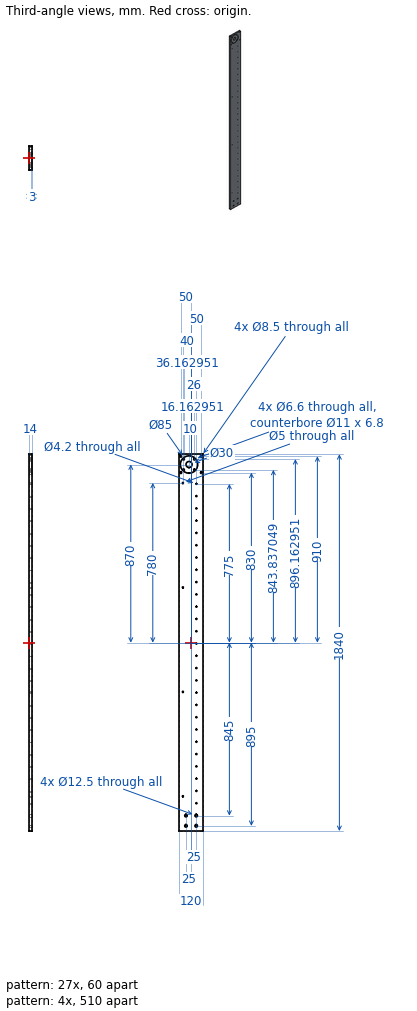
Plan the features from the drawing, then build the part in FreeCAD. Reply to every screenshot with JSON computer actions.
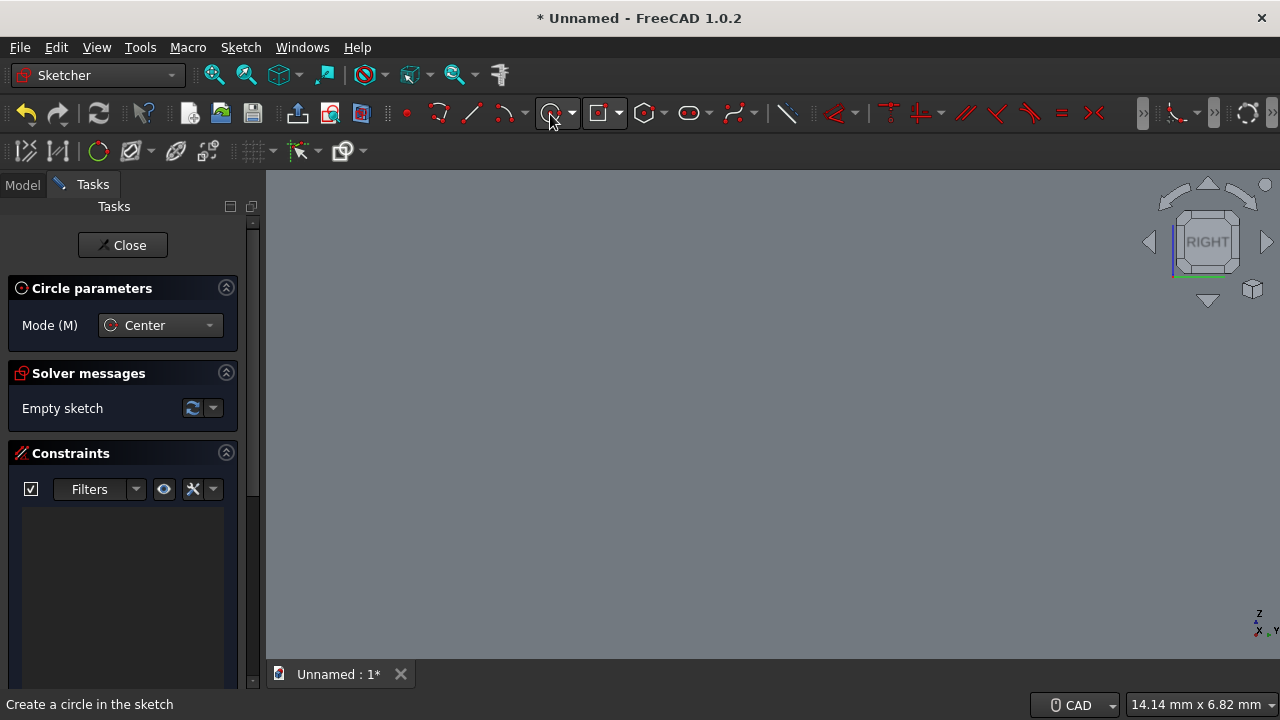
{"action": "left_click", "coordinate": [696, 404]}
{"action": "mouse_move", "coordinate": [803, 297]}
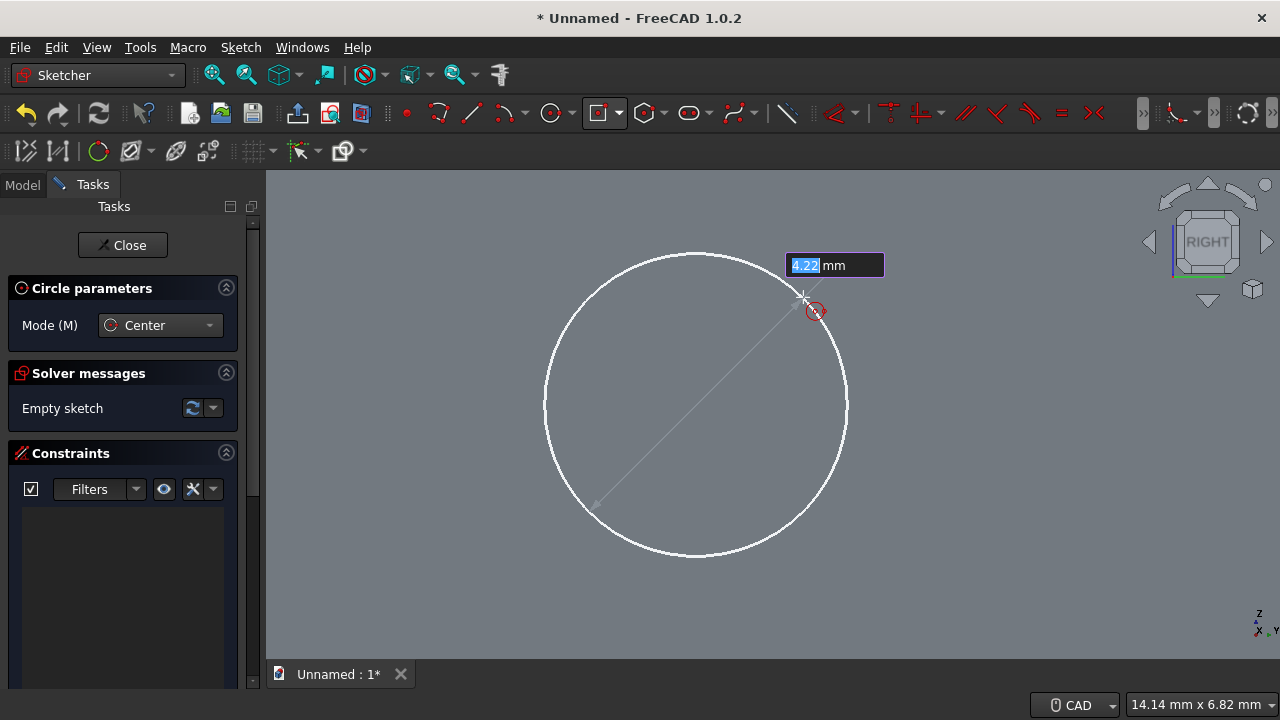
{"action": "type", "text": "4.2"}
{"action": "key", "text": "Return"}
{"action": "key", "text": "Escape"}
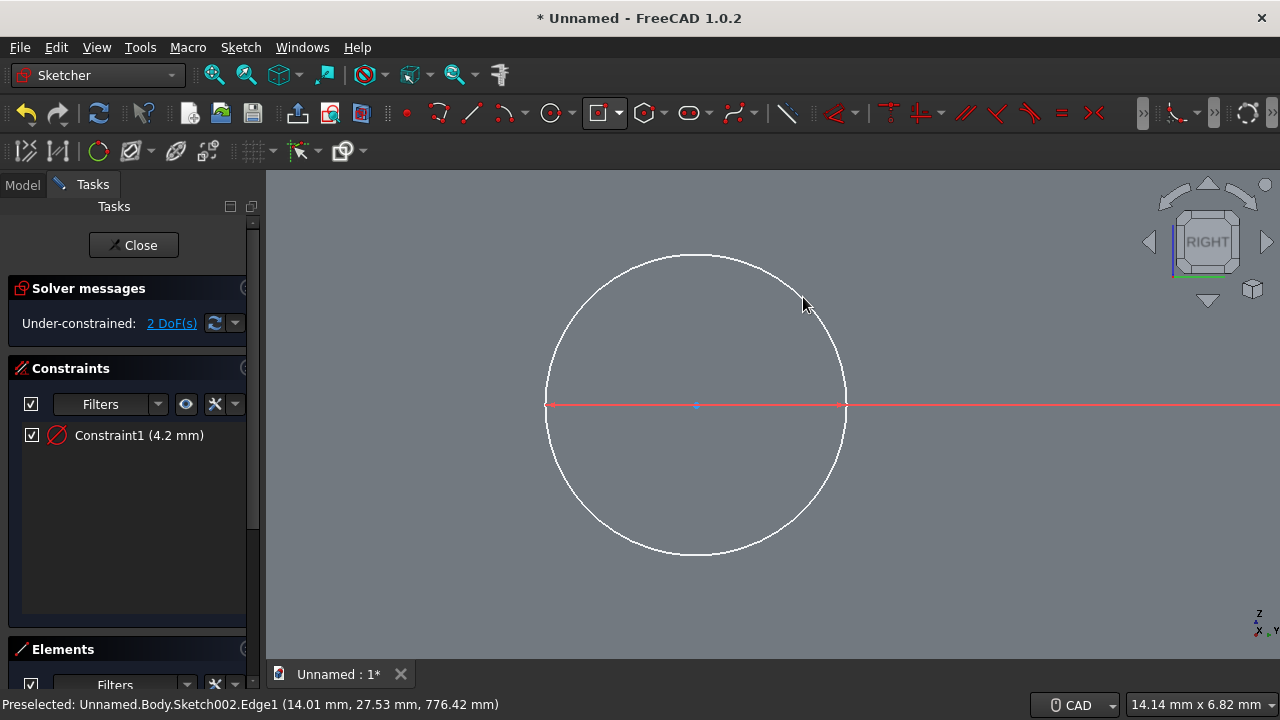
{"action": "left_click", "coordinate": [834, 114]}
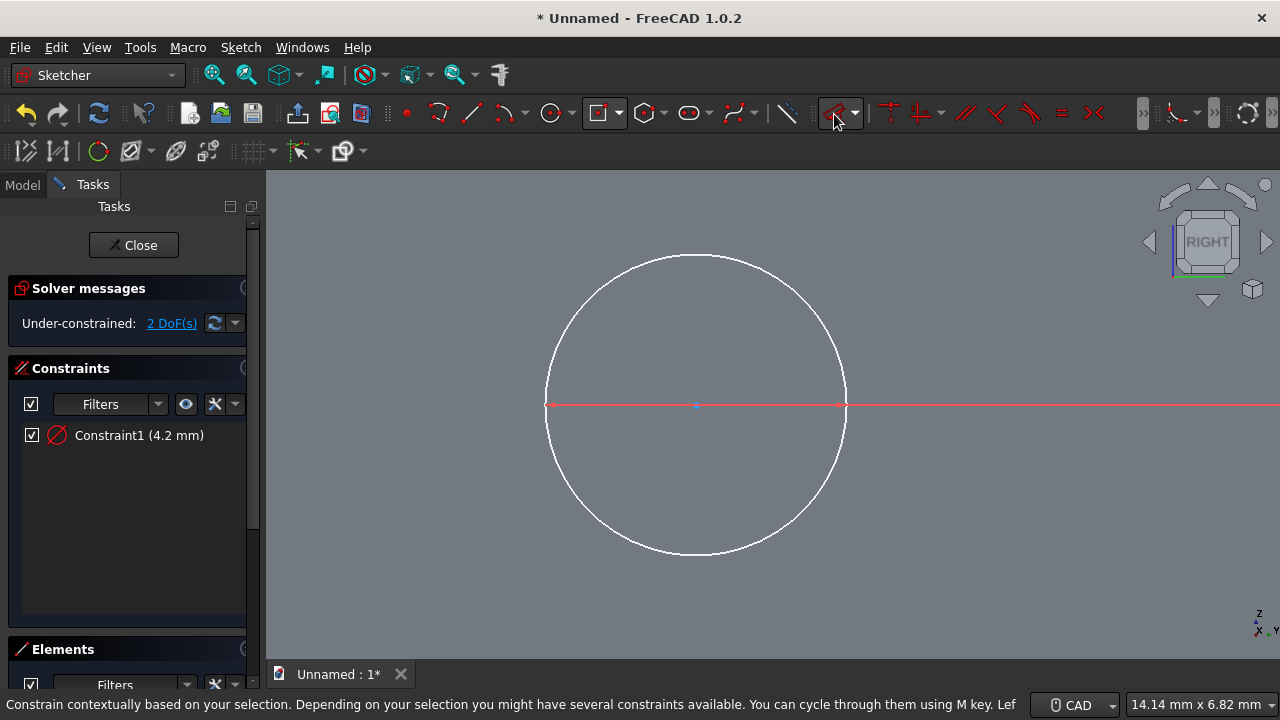
{"action": "left_click", "coordinate": [696, 405]}
{"action": "left_click", "coordinate": [495, 371]}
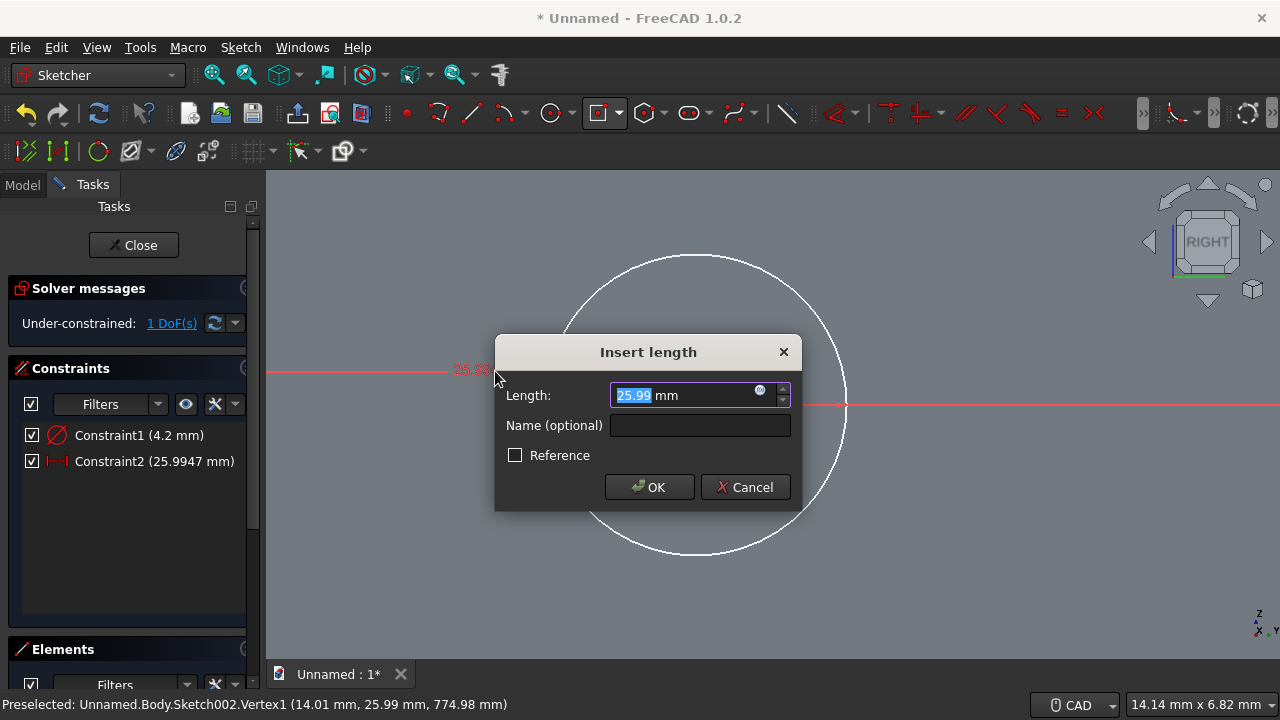
{"action": "type", "text": "26"}
{"action": "key", "text": "Return"}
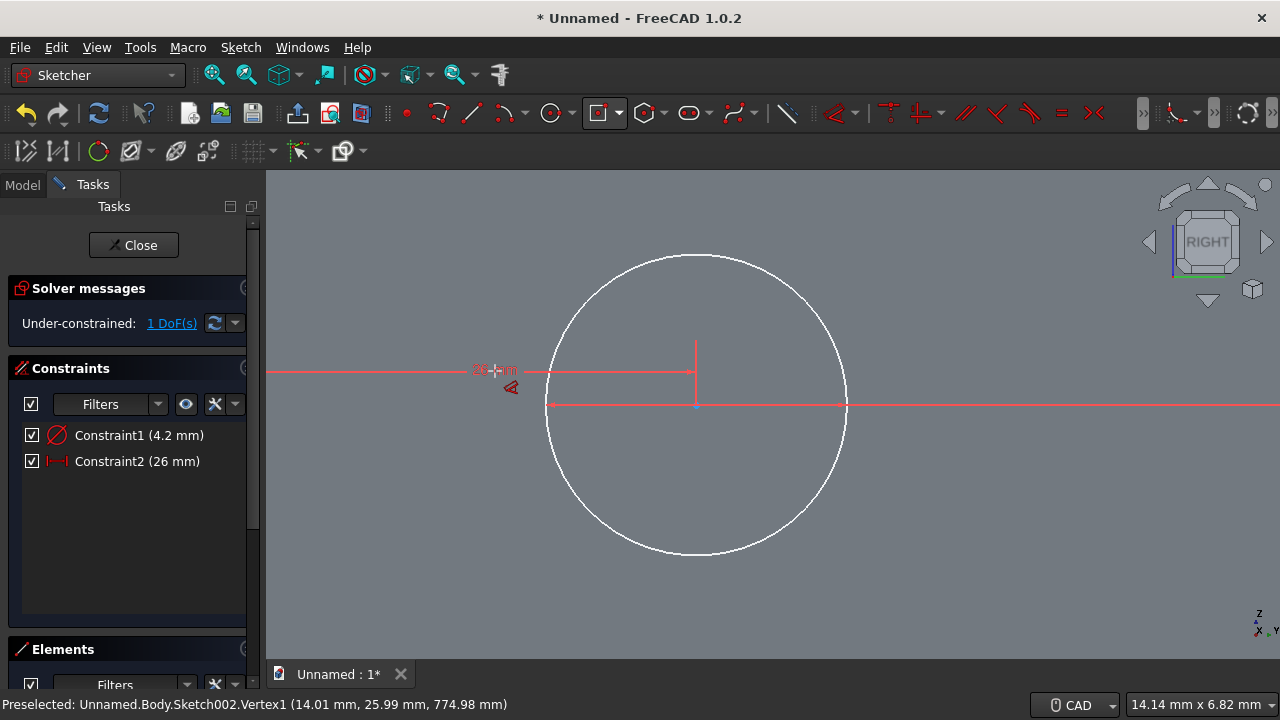
{"action": "left_click", "coordinate": [696, 405]}
{"action": "left_click", "coordinate": [730, 518]}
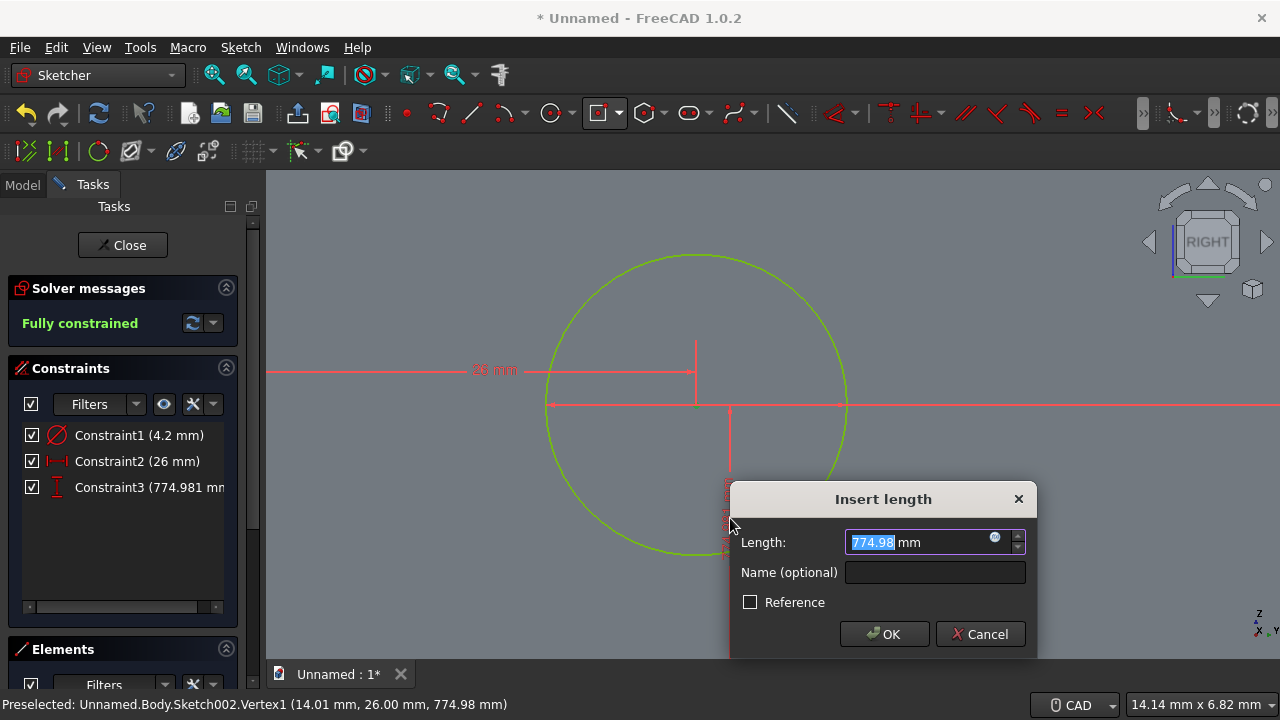
{"action": "type", "text": "775"}
{"action": "key", "text": "Return"}
{"action": "key", "text": "Escape"}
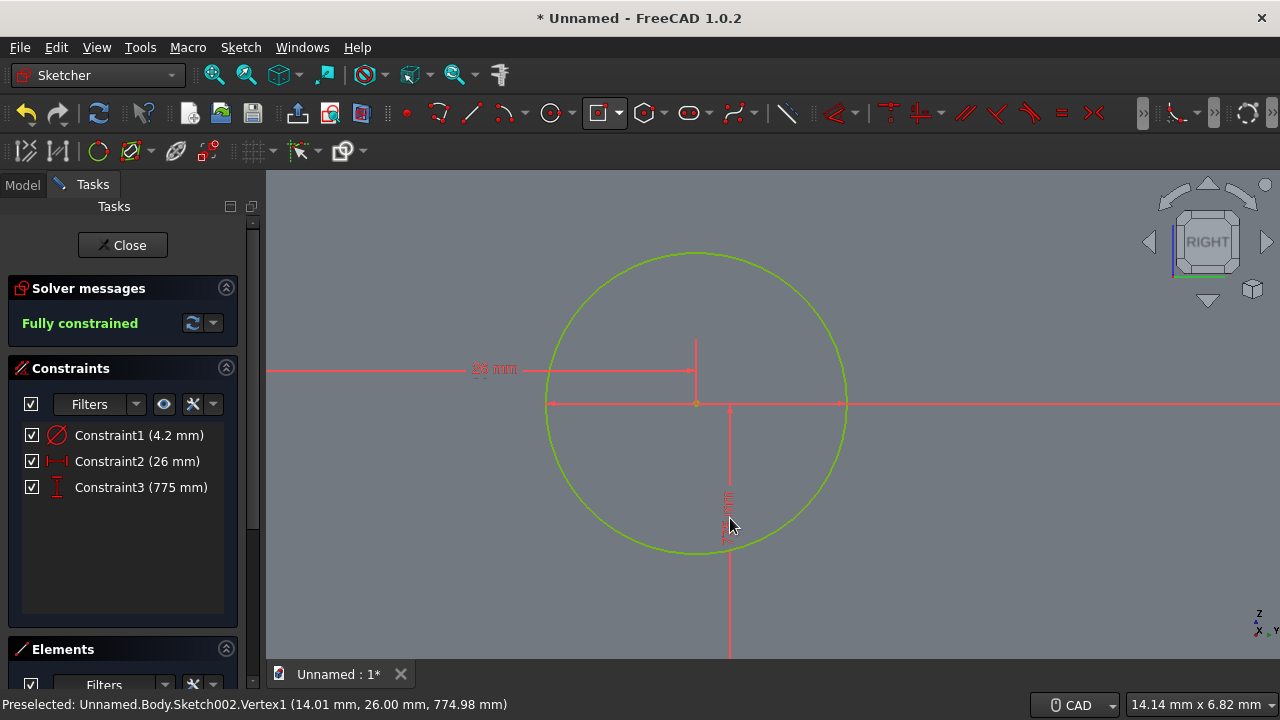
{"action": "left_click", "coordinate": [123, 245]}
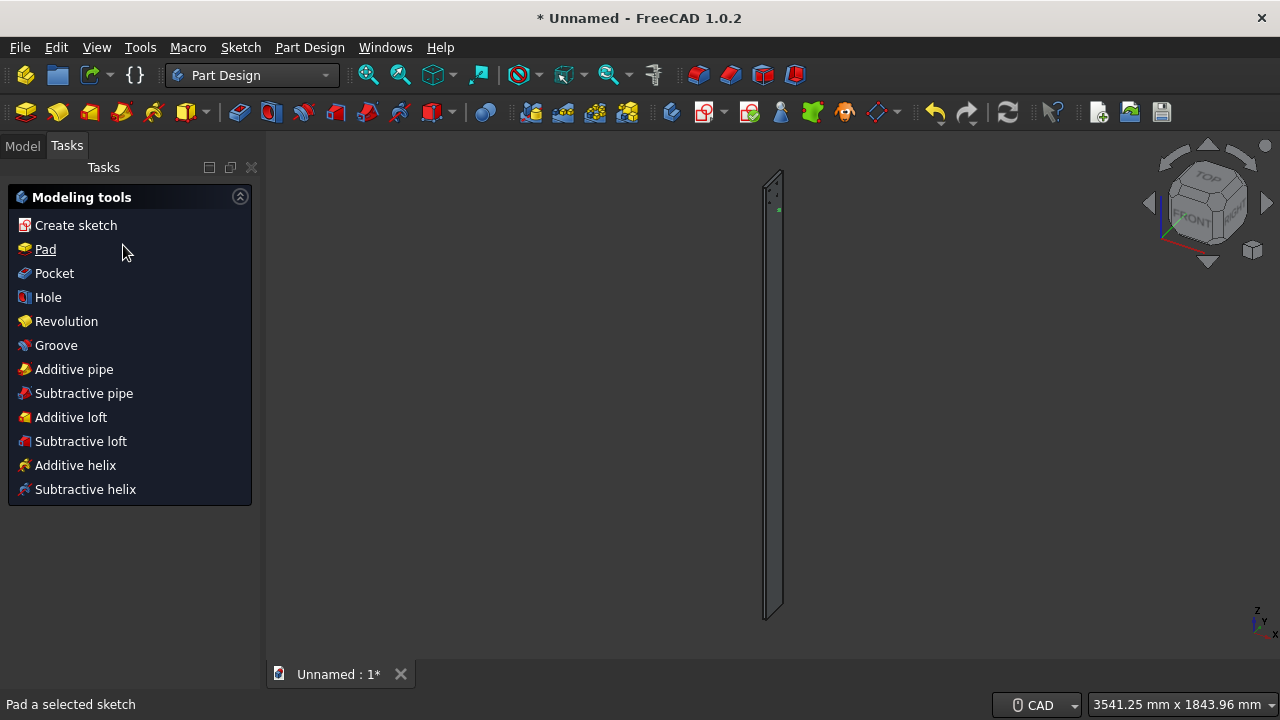
{"action": "left_click", "coordinate": [272, 112]}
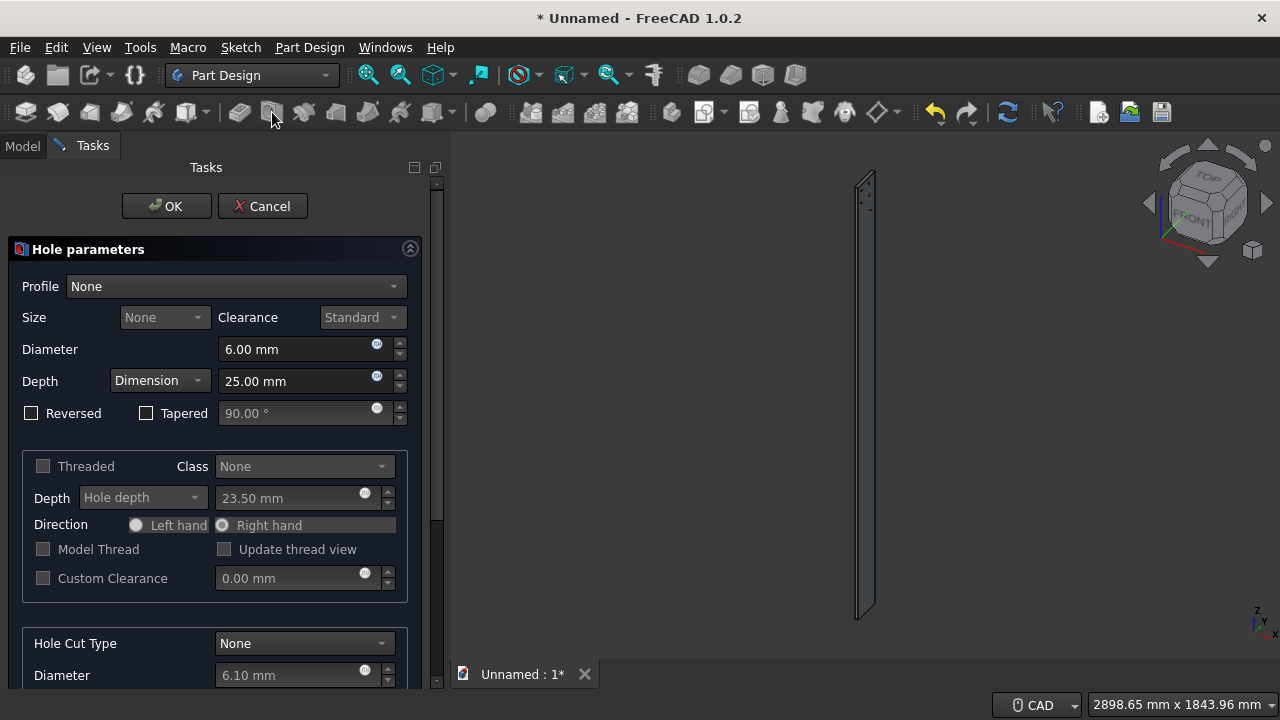
{"action": "triple_click", "coordinate": [305, 349]}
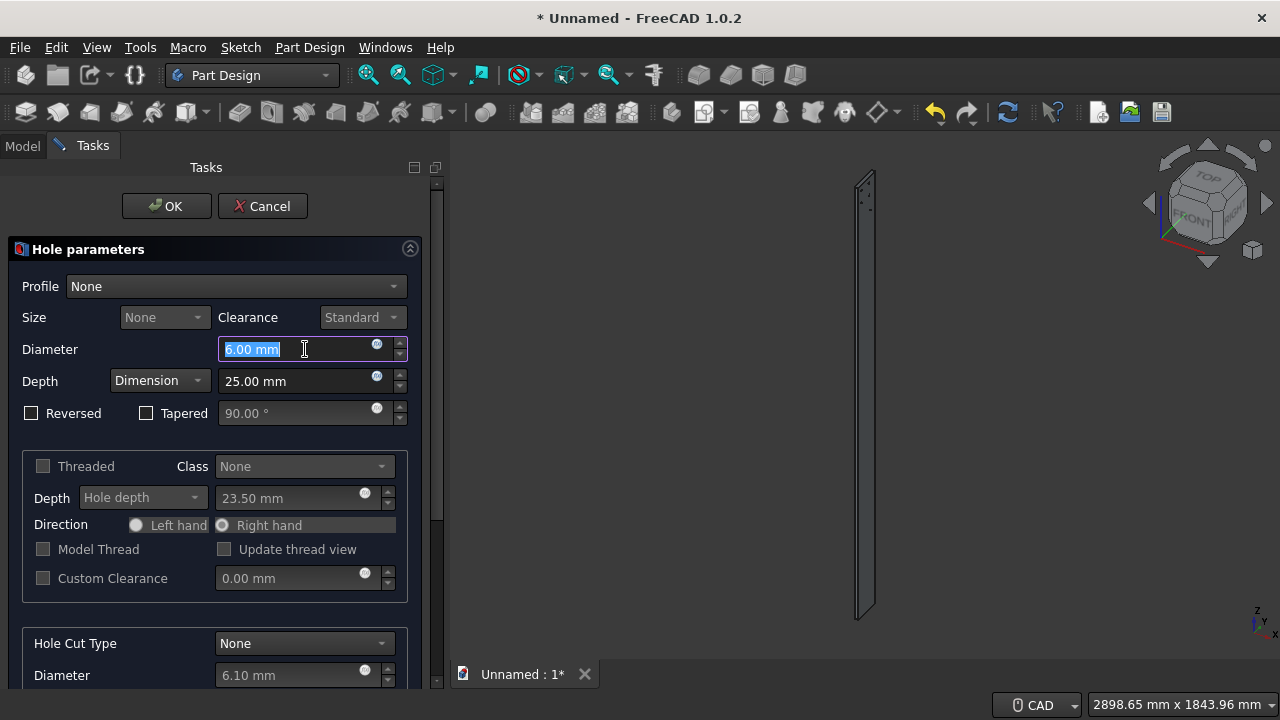
{"action": "type", "text": "4.2"}
{"action": "key", "text": "Tab"}